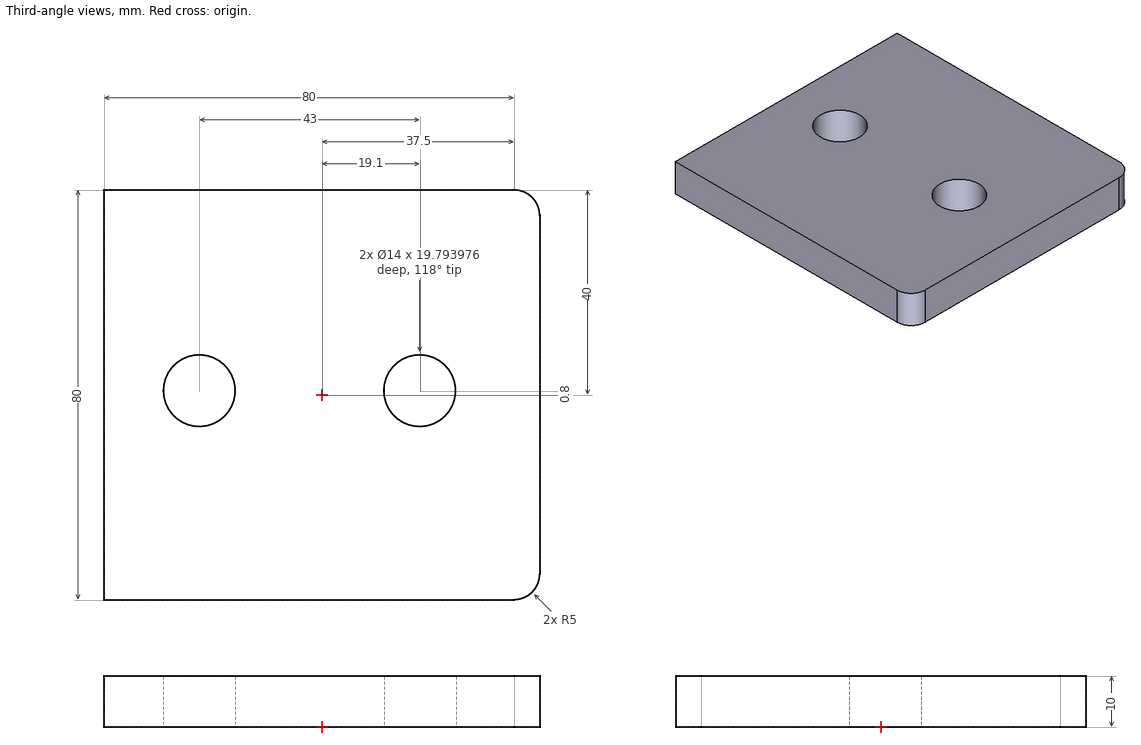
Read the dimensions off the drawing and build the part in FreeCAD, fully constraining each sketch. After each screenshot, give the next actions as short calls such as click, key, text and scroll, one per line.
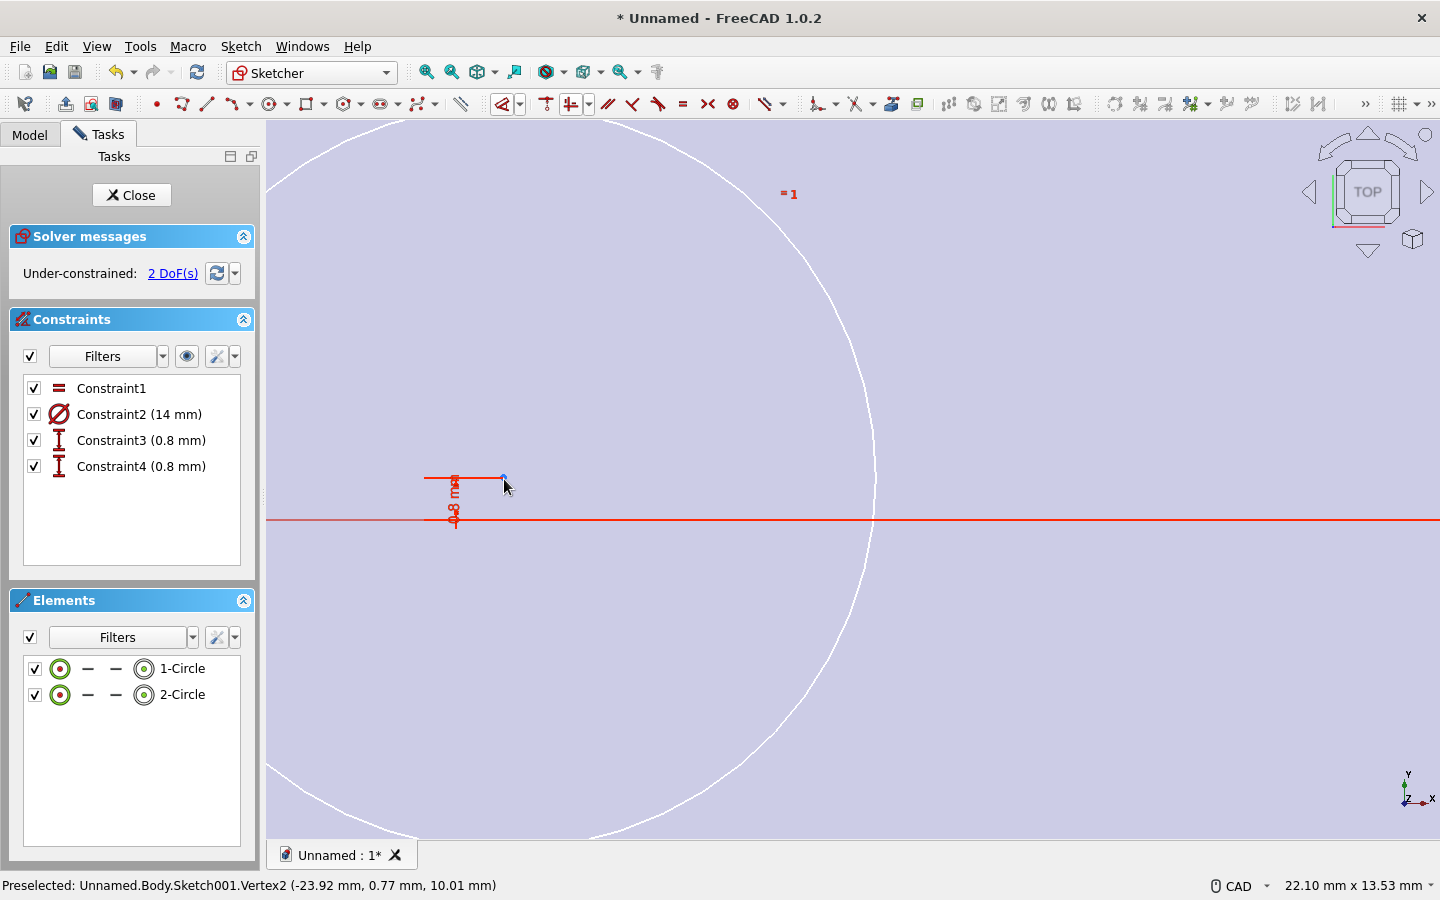
scroll(502, 480, down, 7)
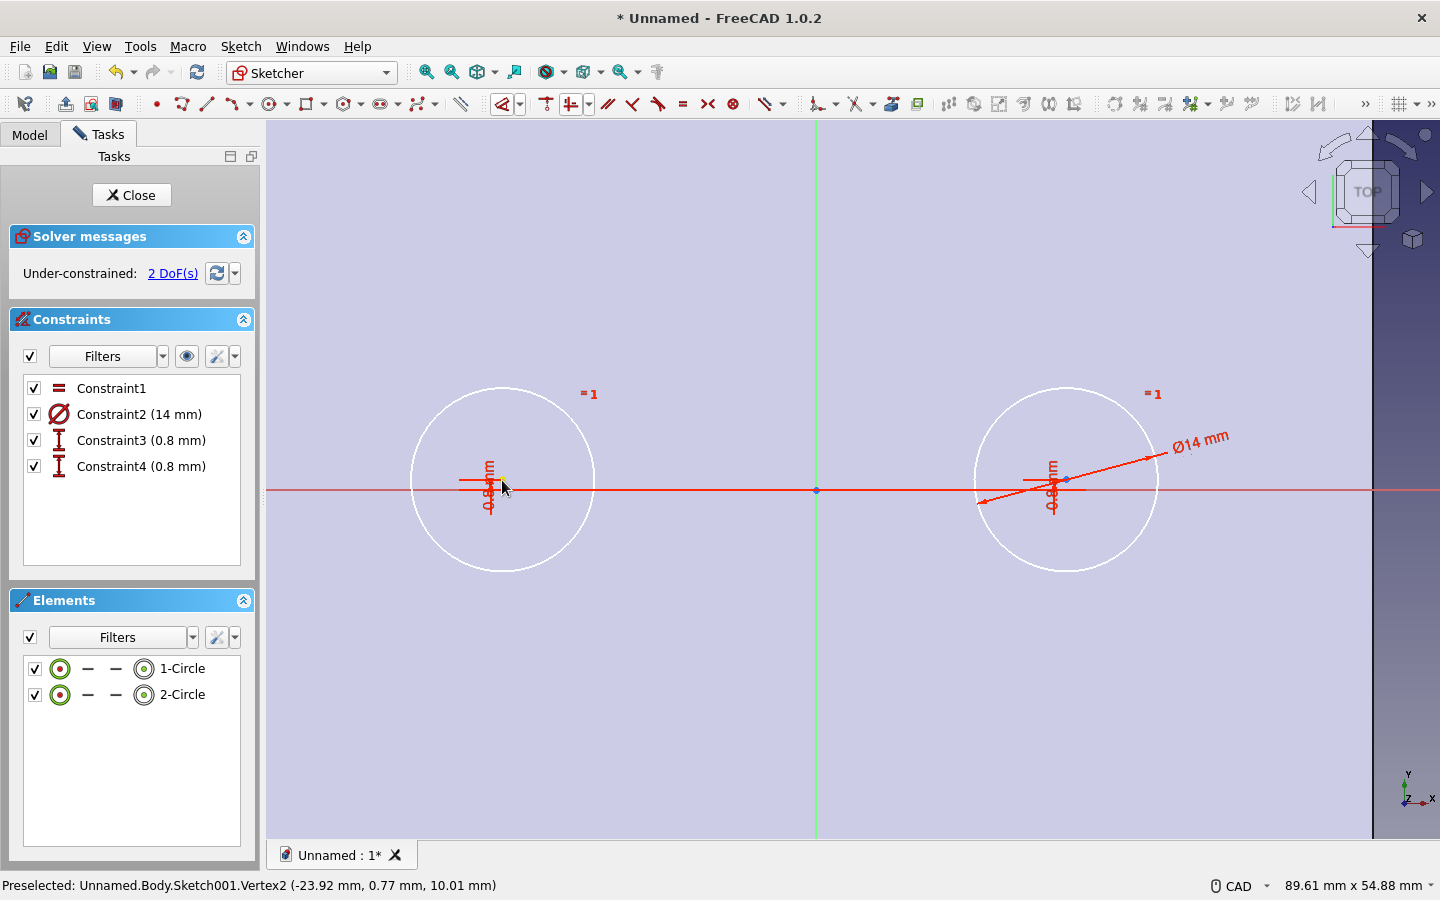
click(1066, 480)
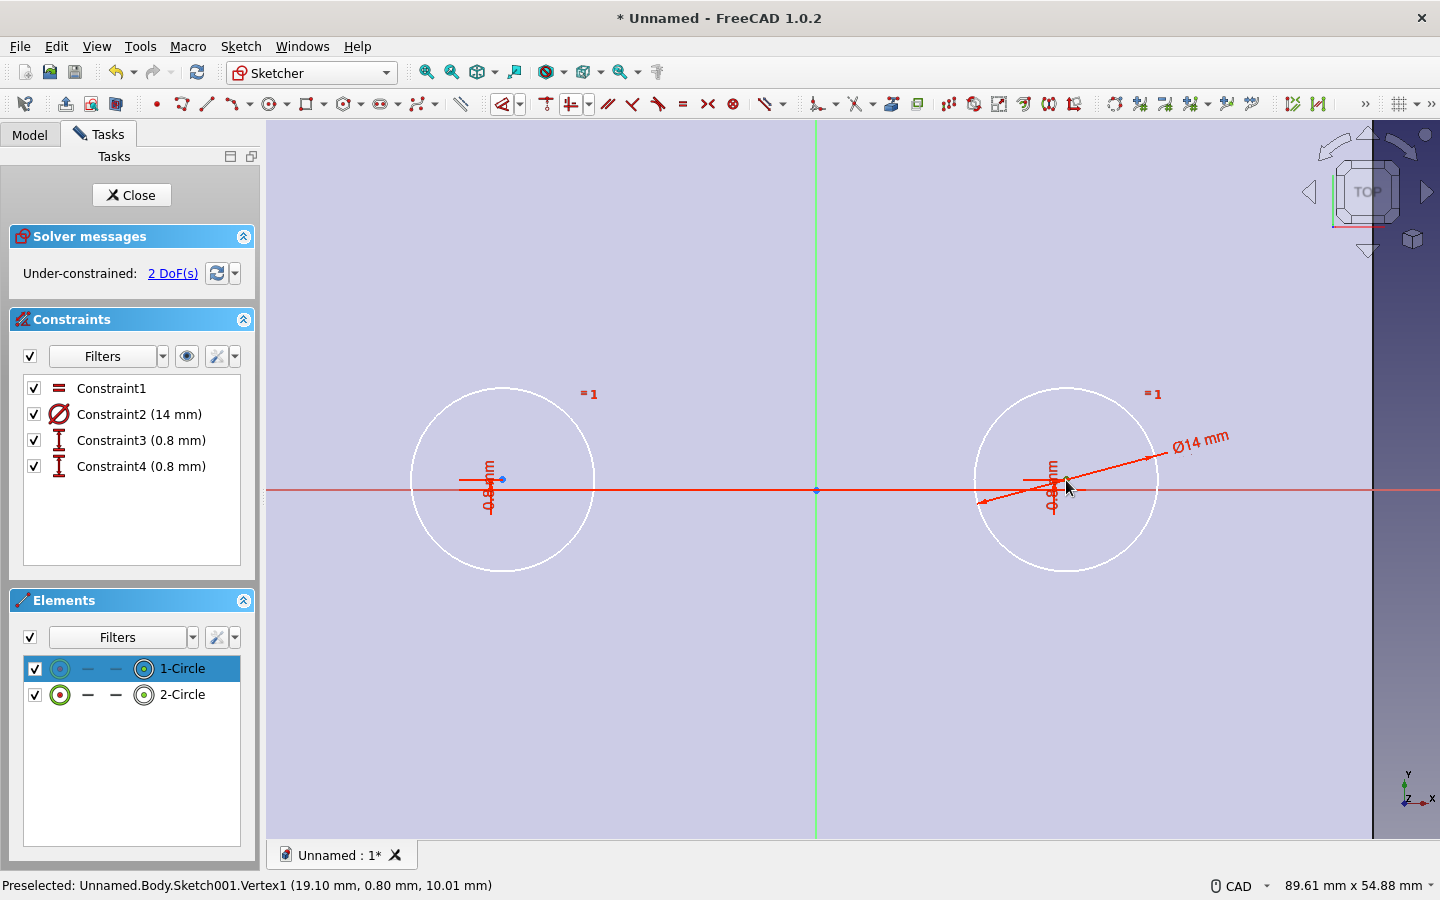
click(503, 480)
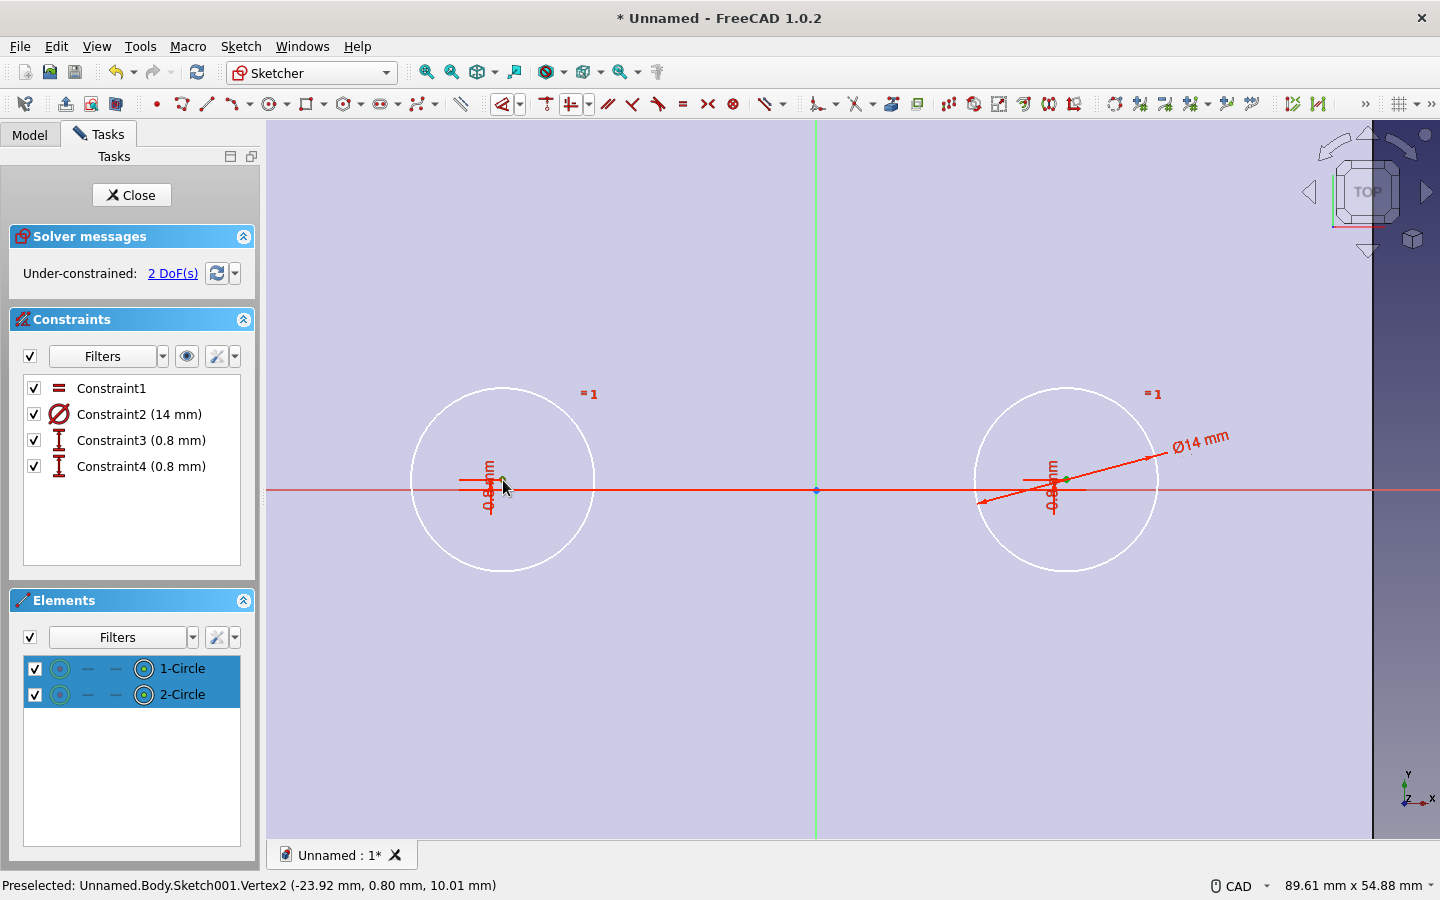
click(520, 104)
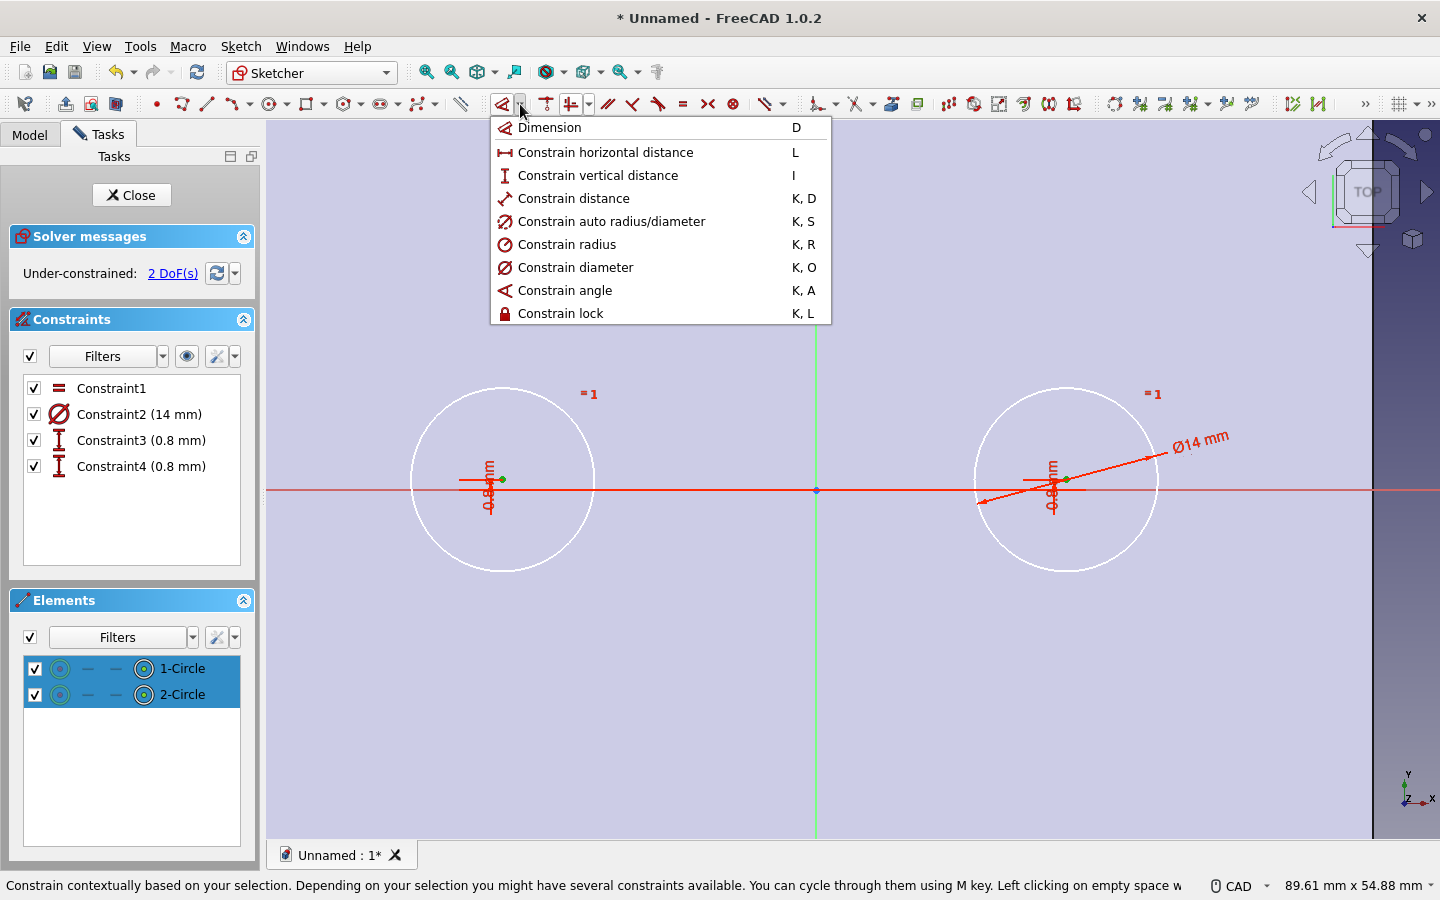
click(661, 152)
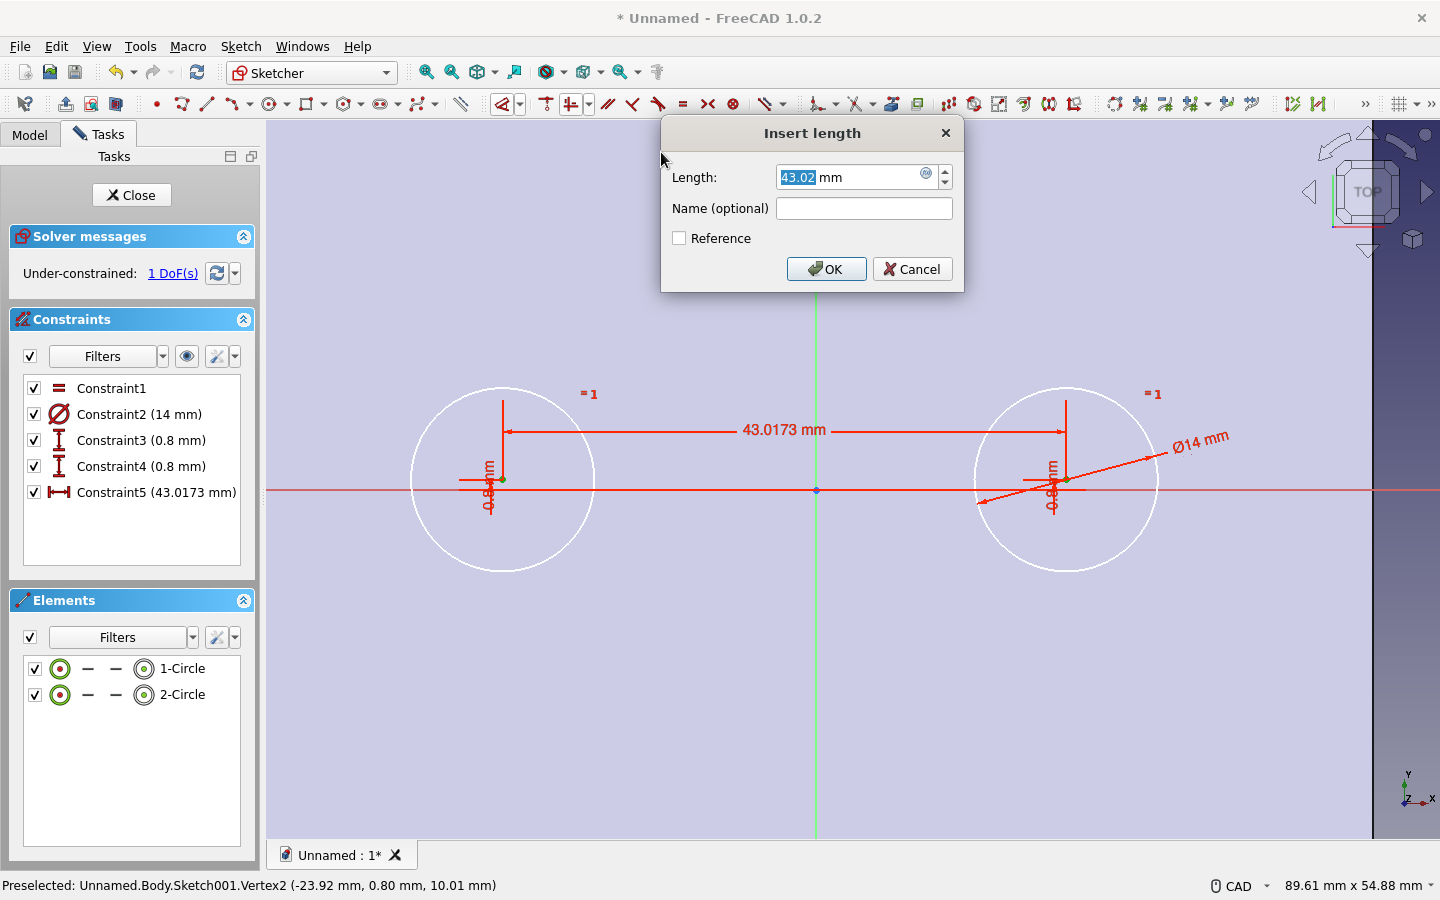
text(43)
key(Return)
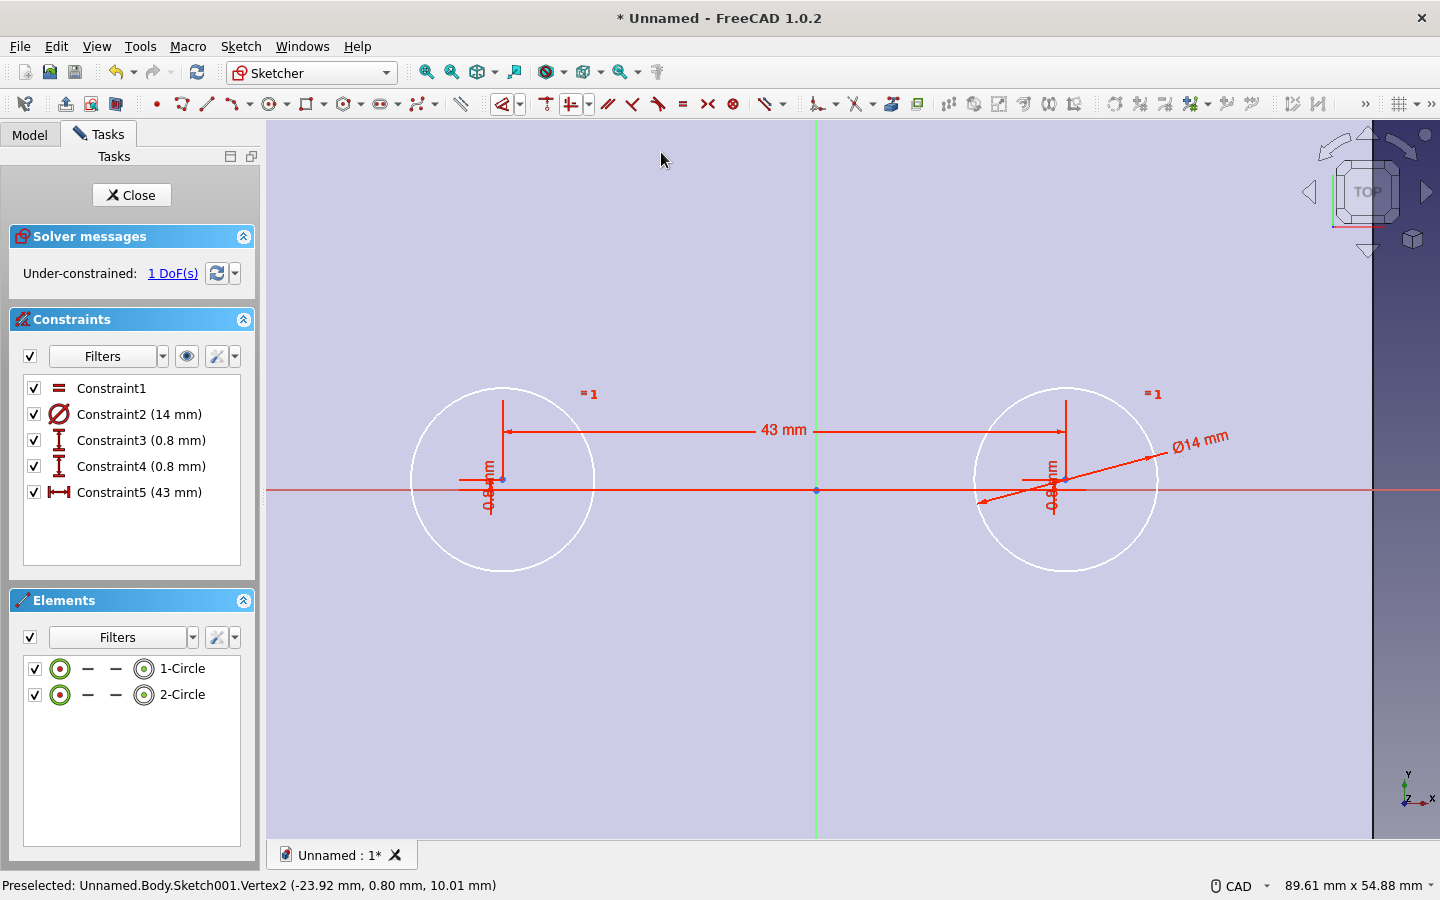
click(1066, 480)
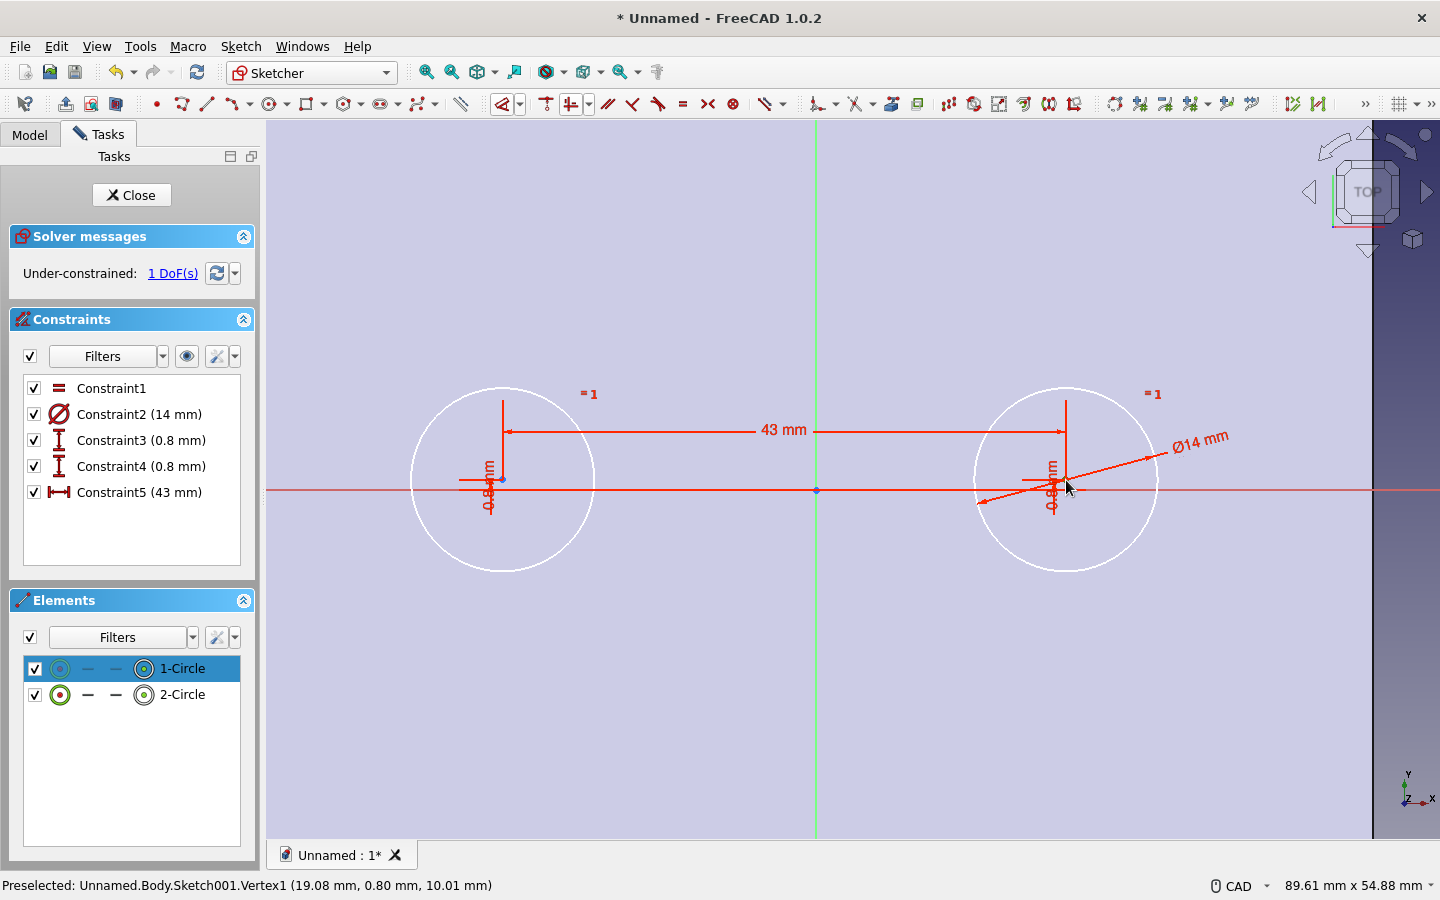
key(l)